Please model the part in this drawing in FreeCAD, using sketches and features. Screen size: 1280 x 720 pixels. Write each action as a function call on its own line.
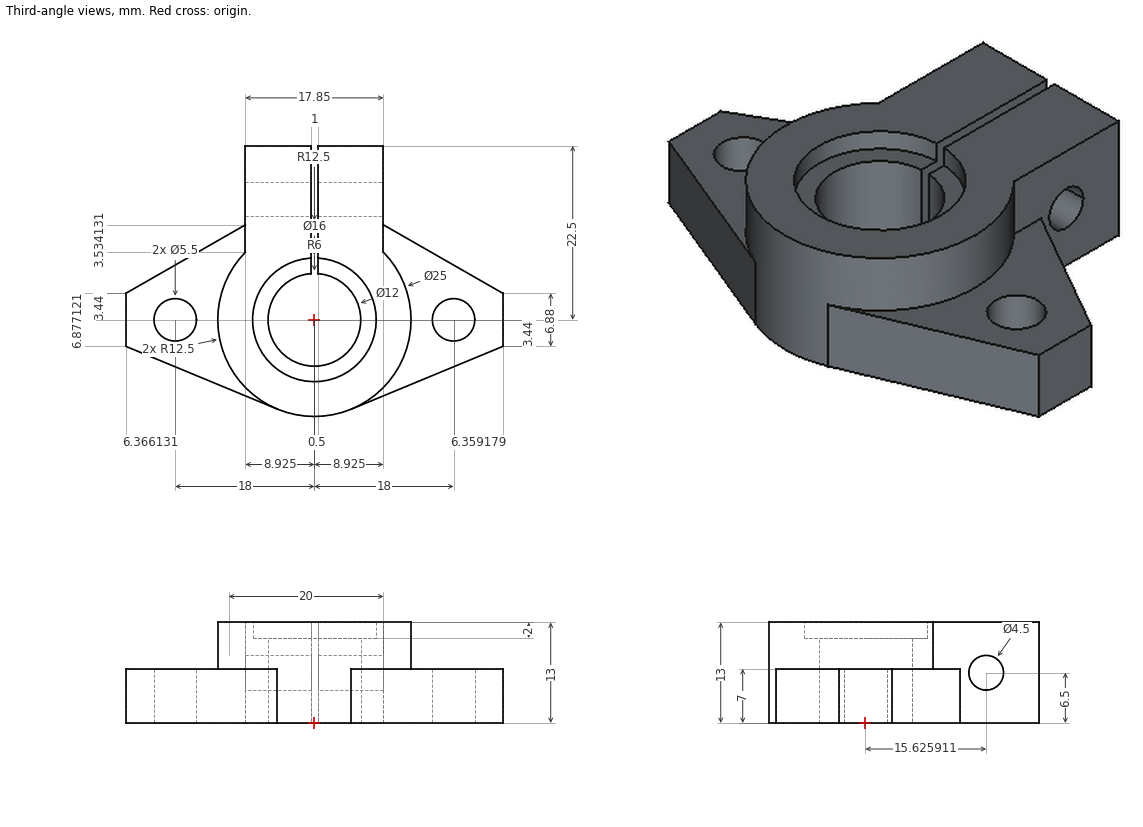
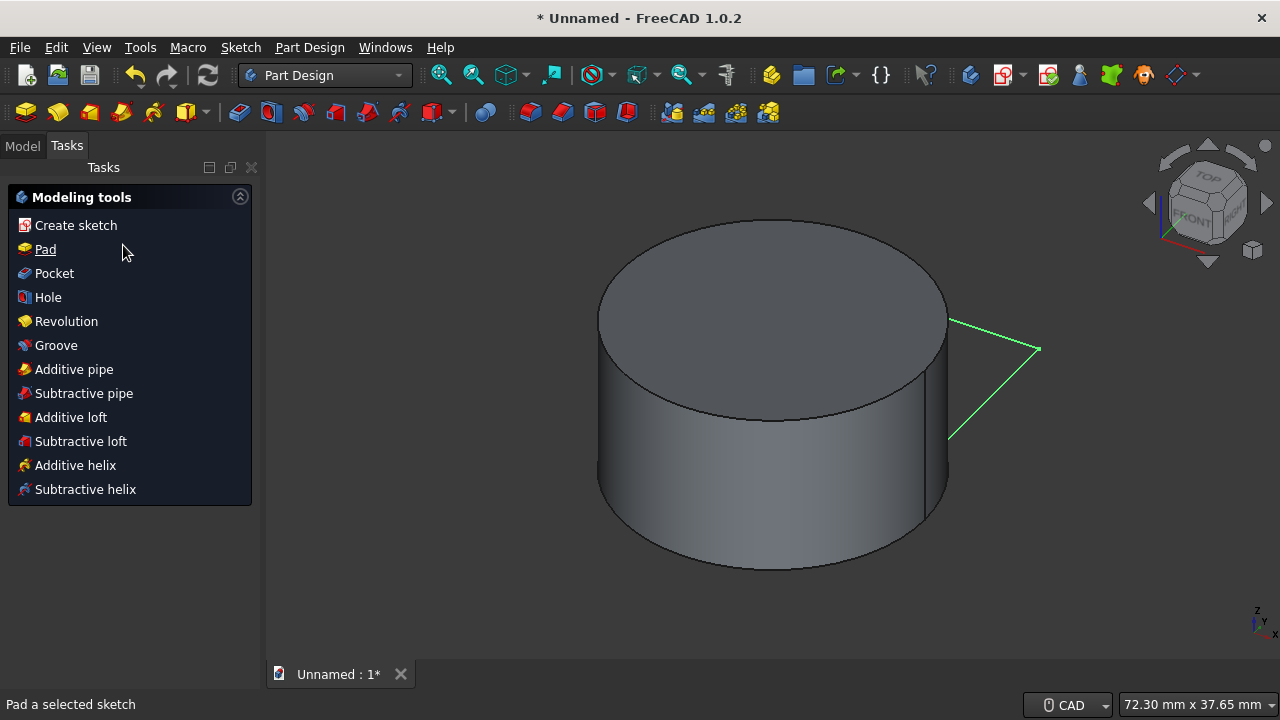
click(26, 112)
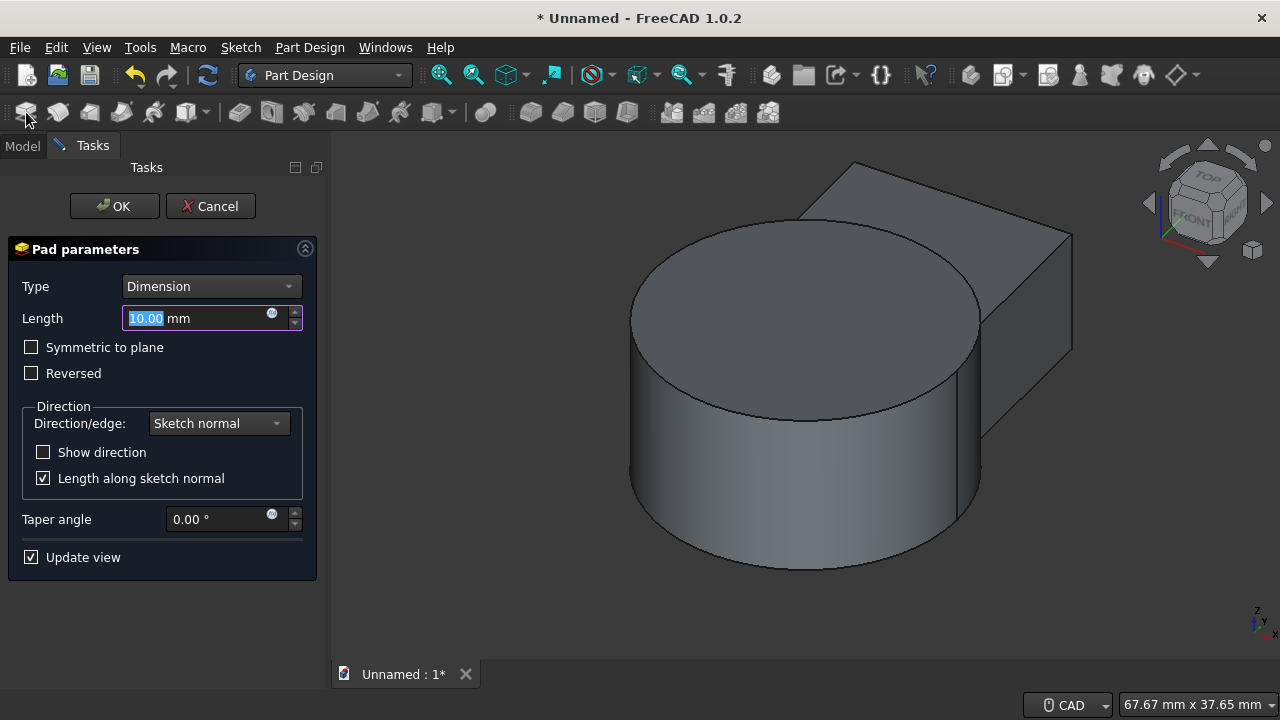
text(13)
key(Tab)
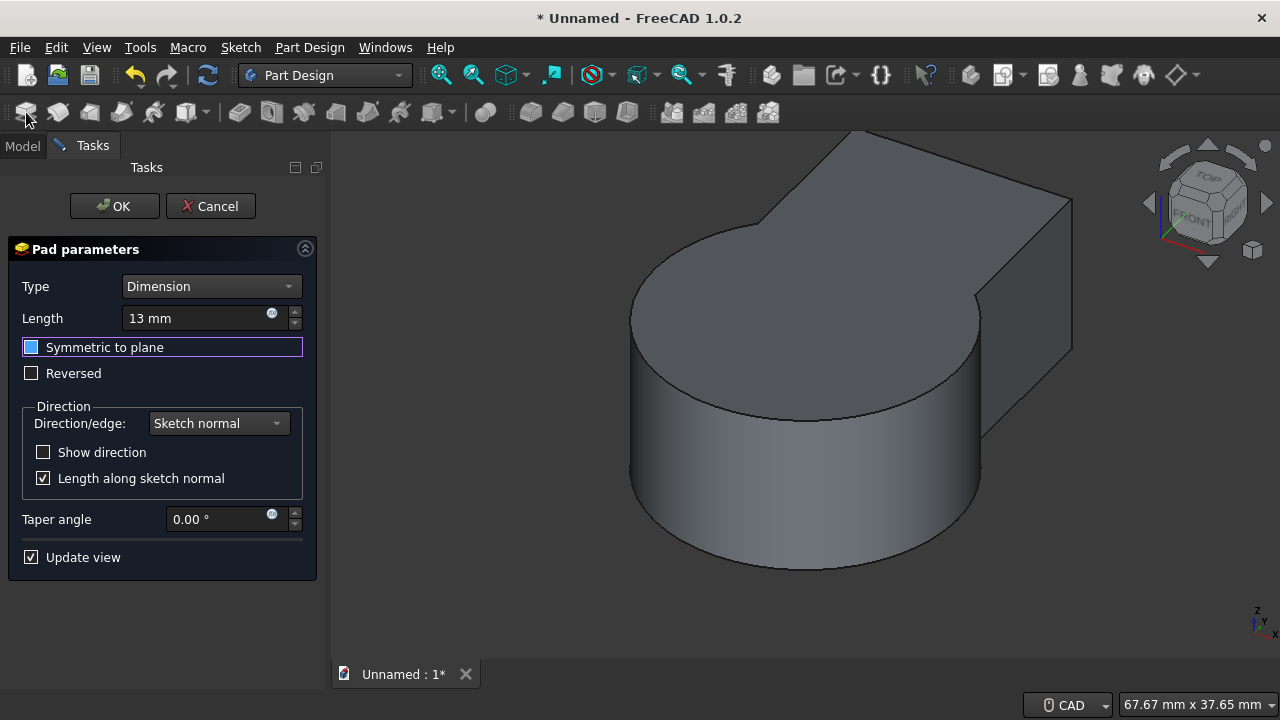
click(115, 206)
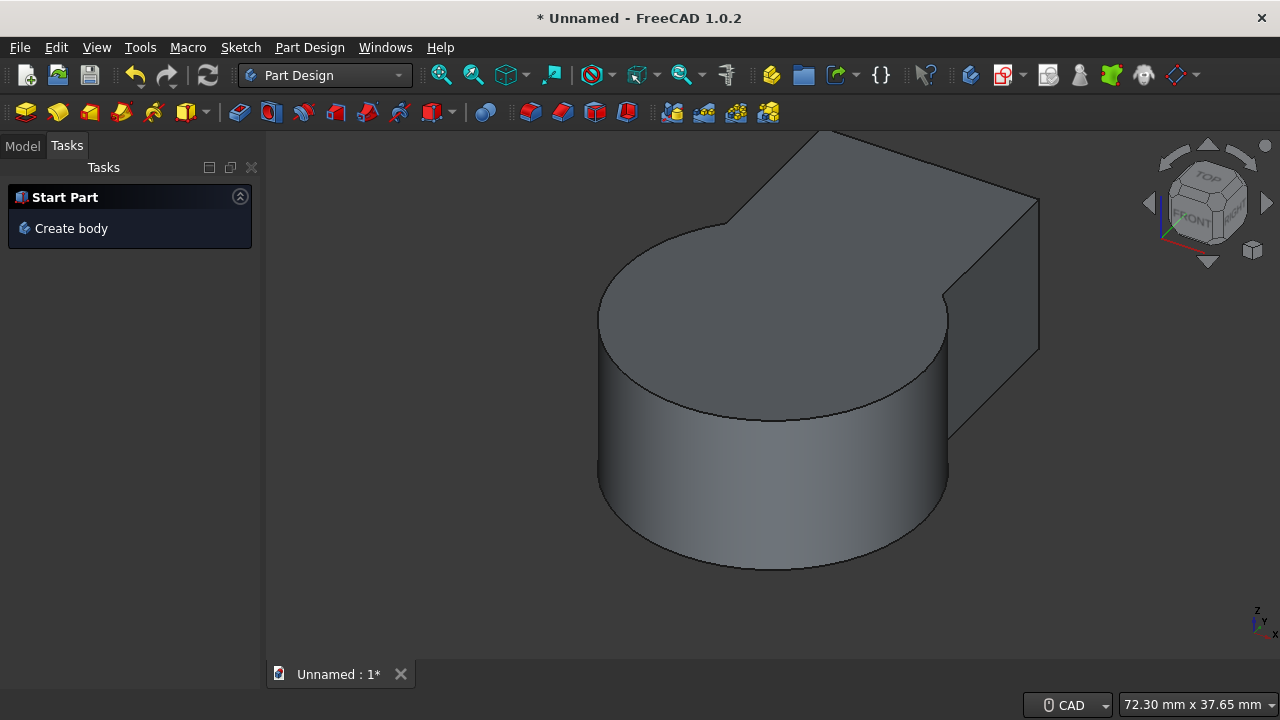
click(442, 76)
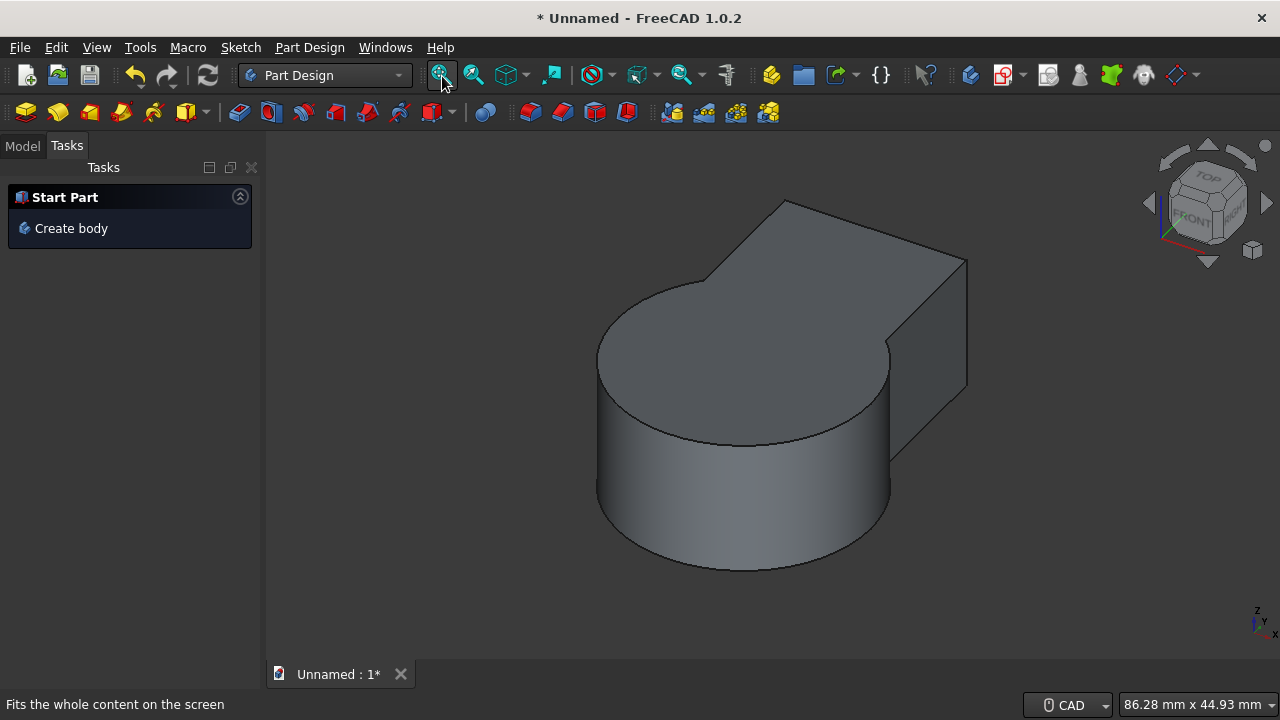
click(744, 361)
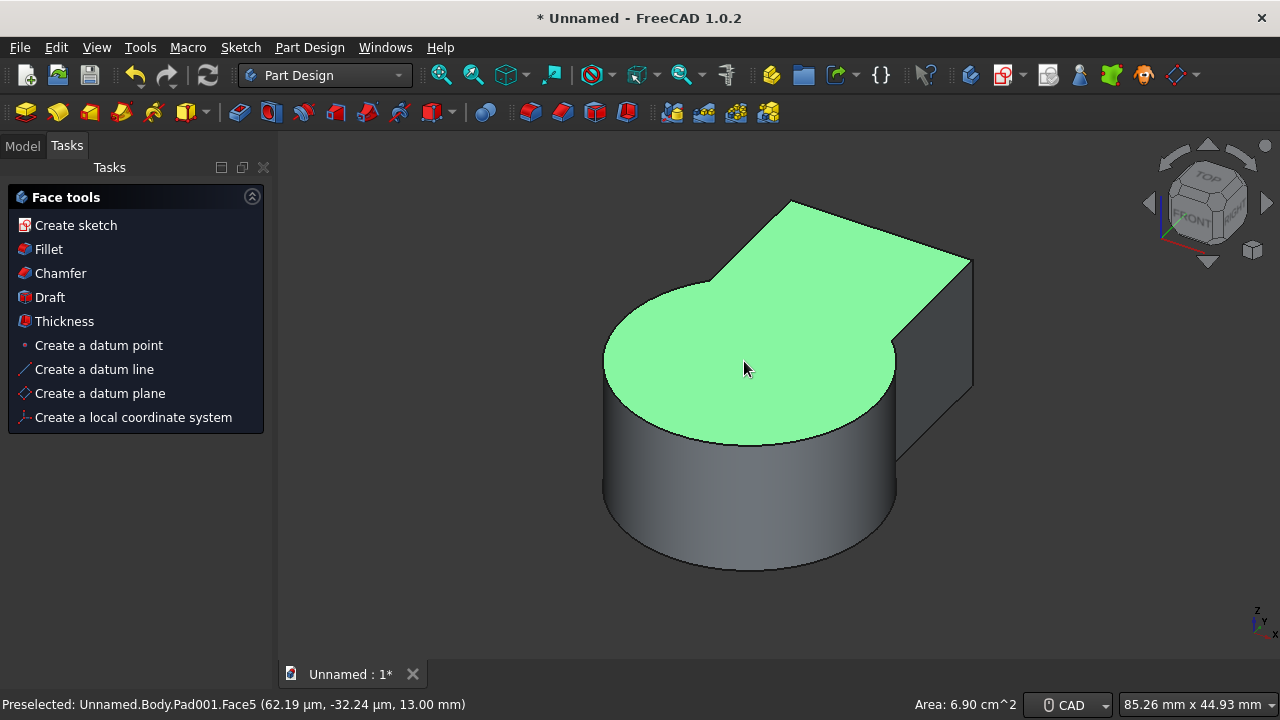
click(1004, 76)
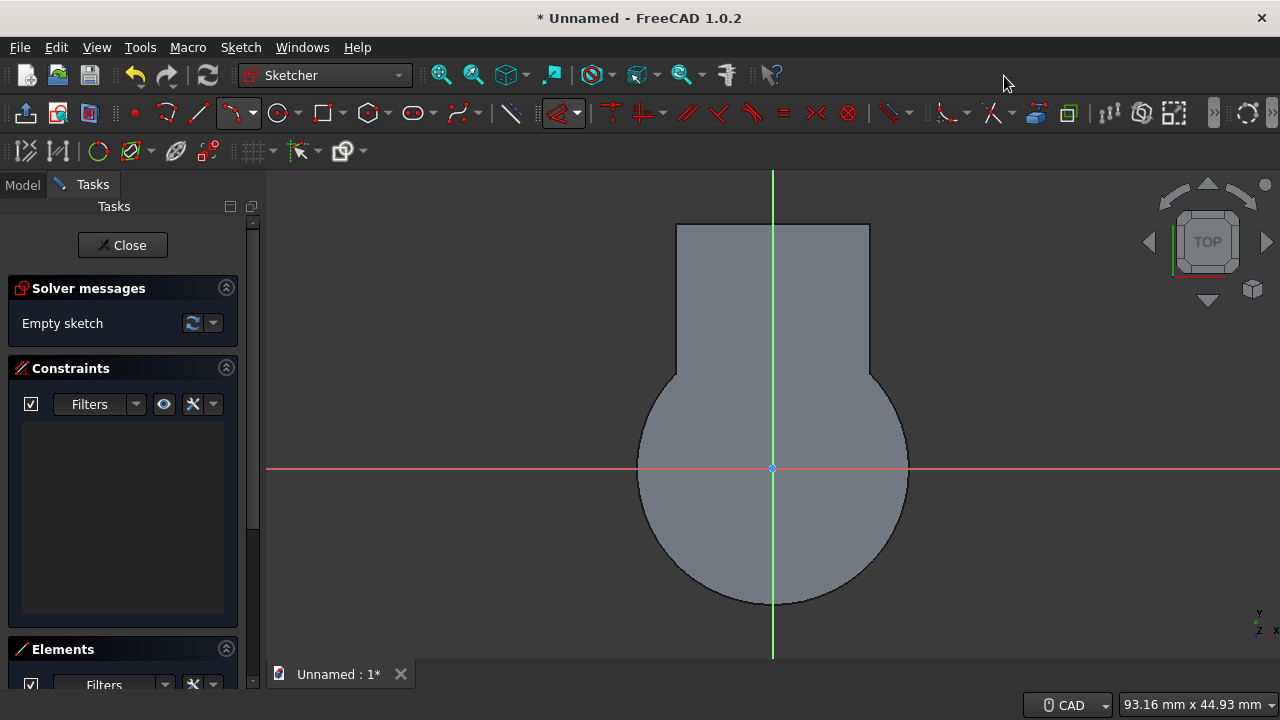
scroll(829, 513, up, 4)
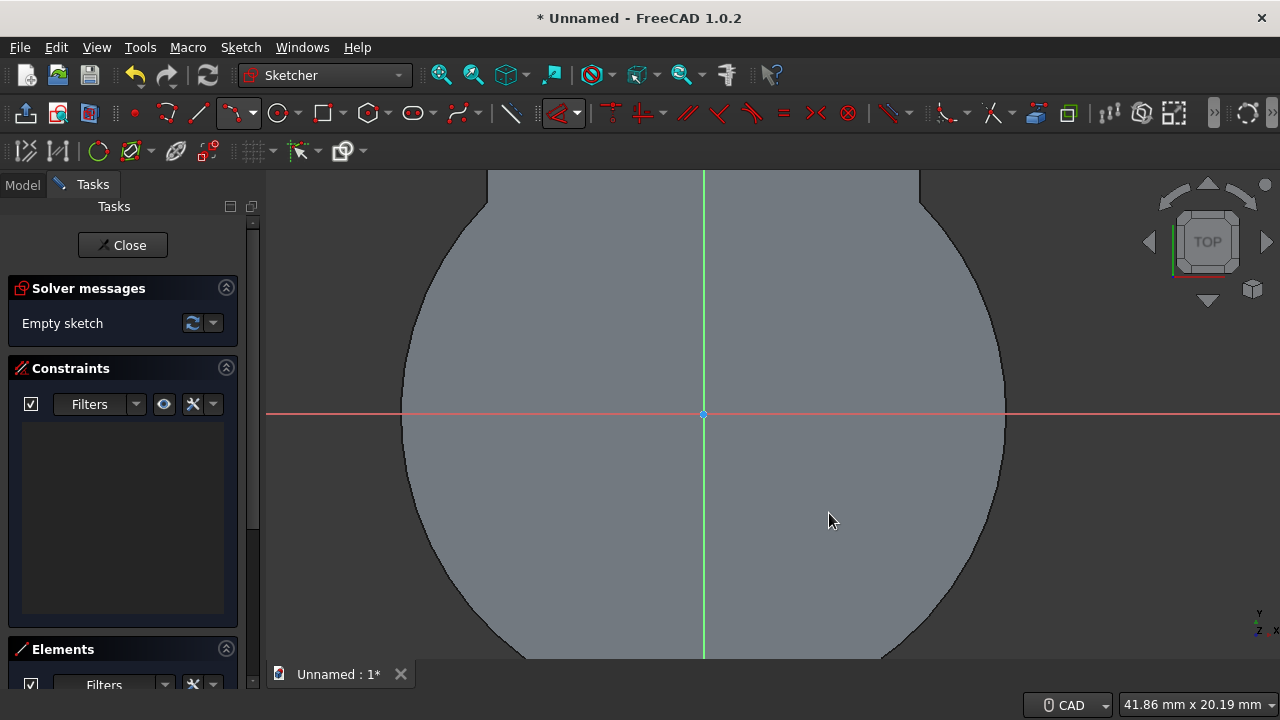
click(278, 114)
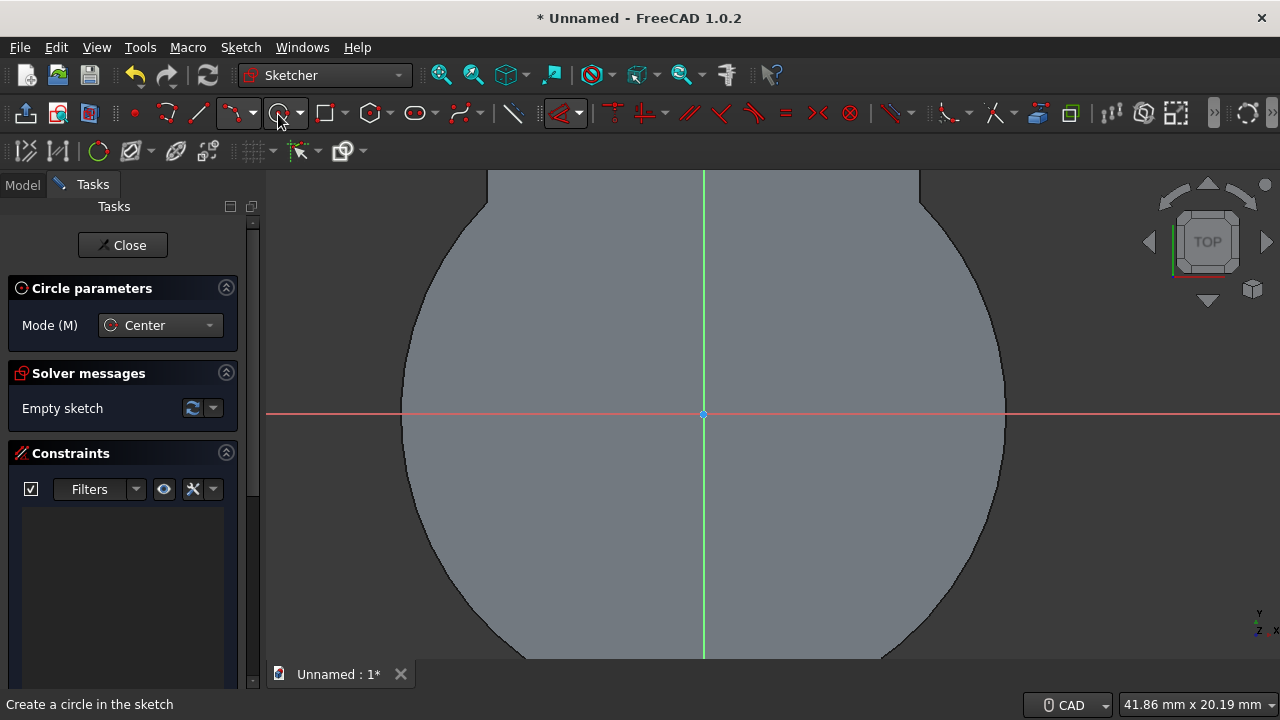
click(704, 414)
click(806, 311)
key(Escape)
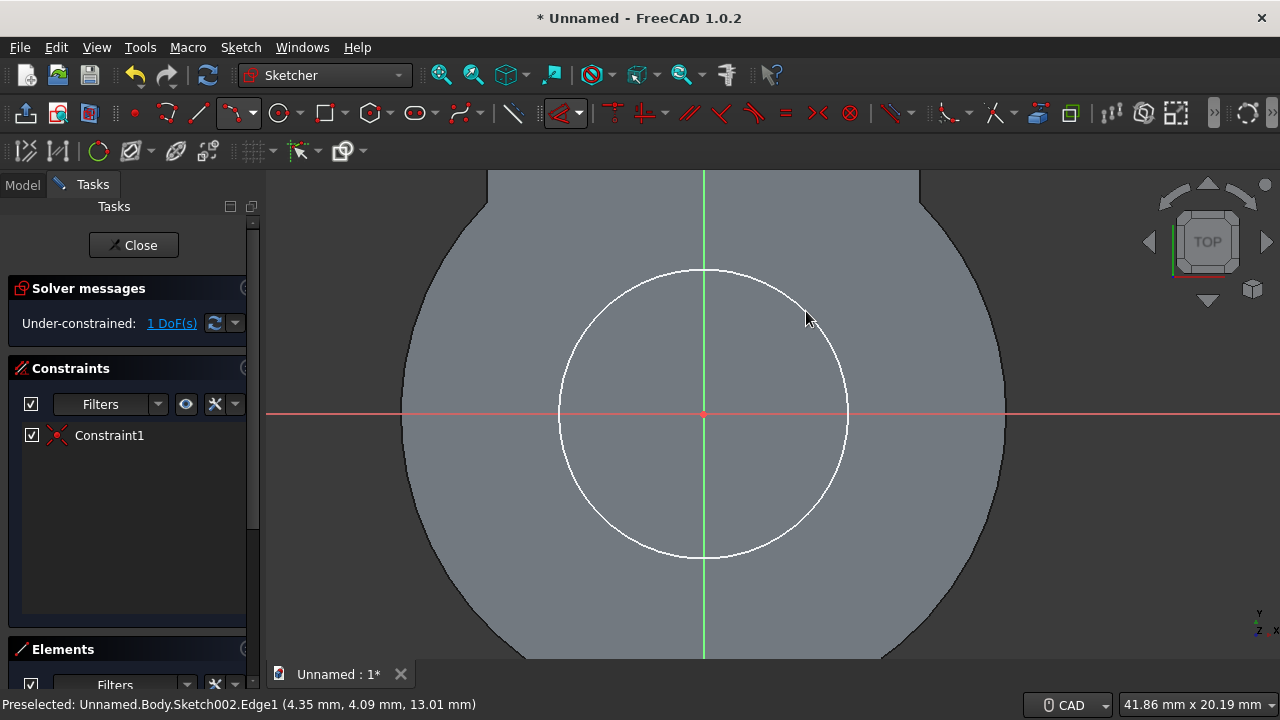
click(806, 312)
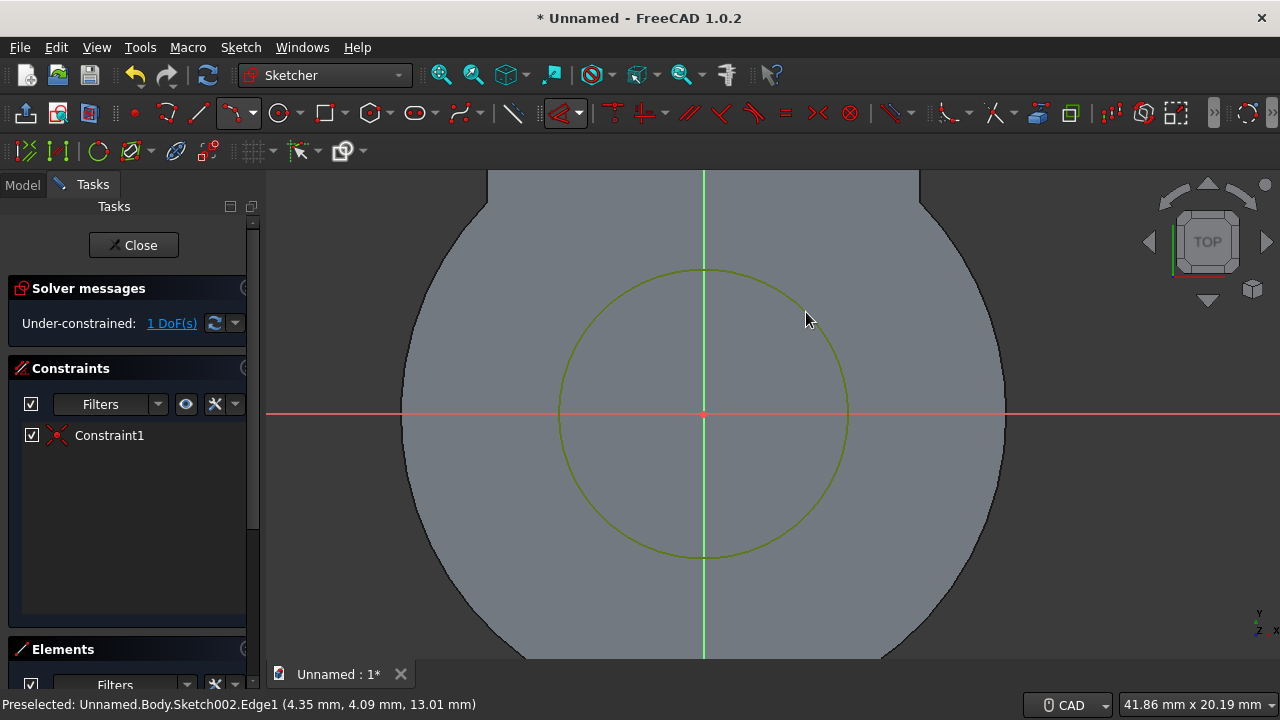
key(k)
key(o)